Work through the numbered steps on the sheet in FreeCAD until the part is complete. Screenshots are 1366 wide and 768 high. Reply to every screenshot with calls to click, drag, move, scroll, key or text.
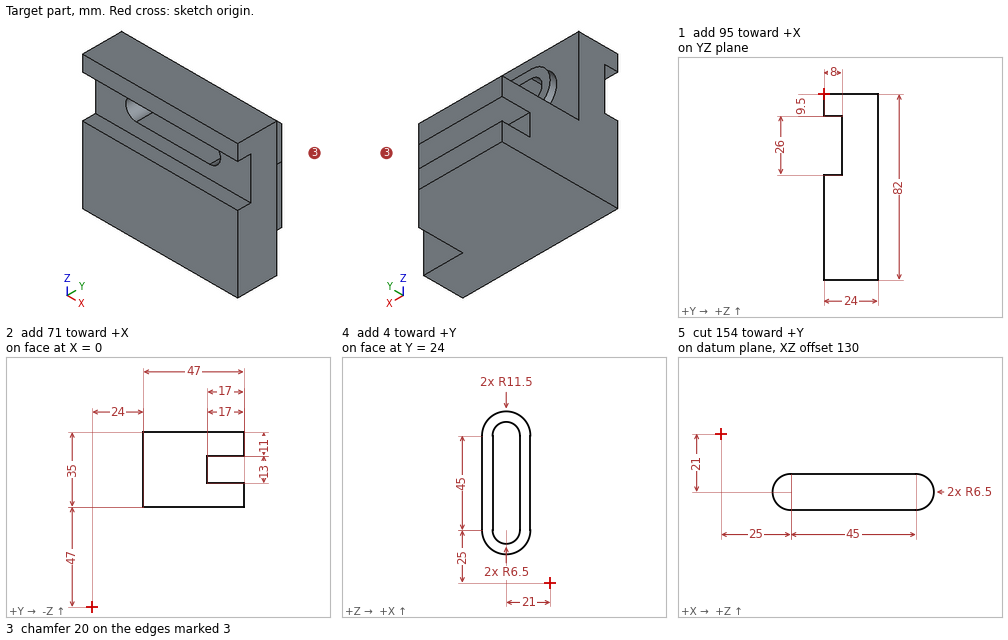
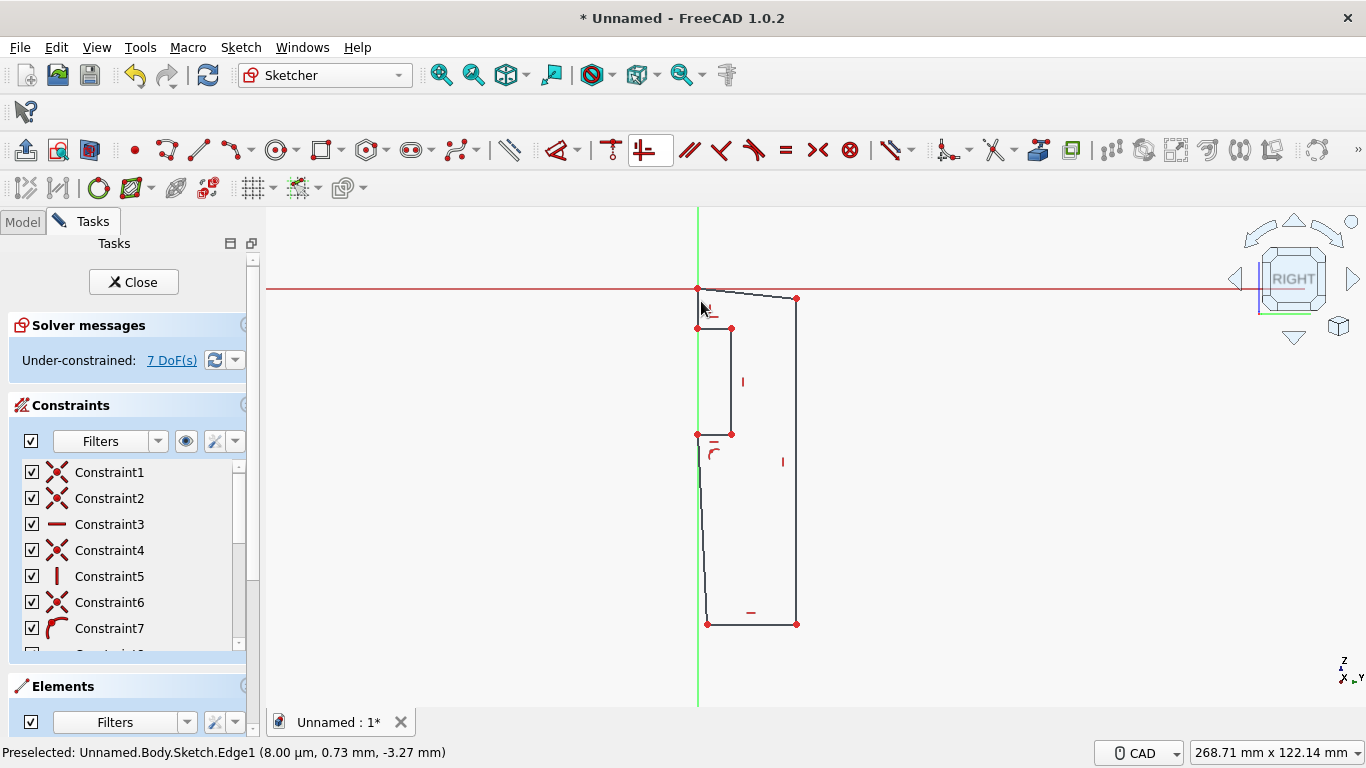
click(701, 492)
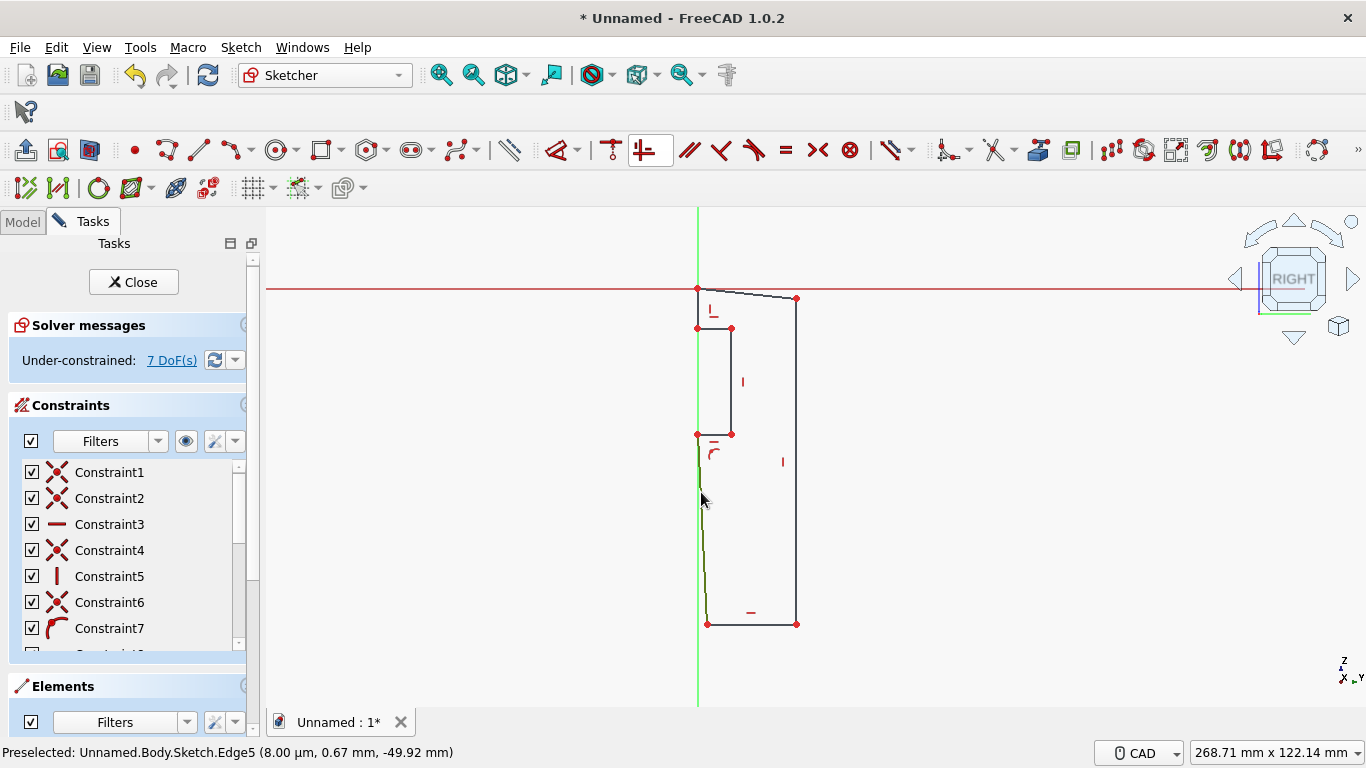
click(668, 150)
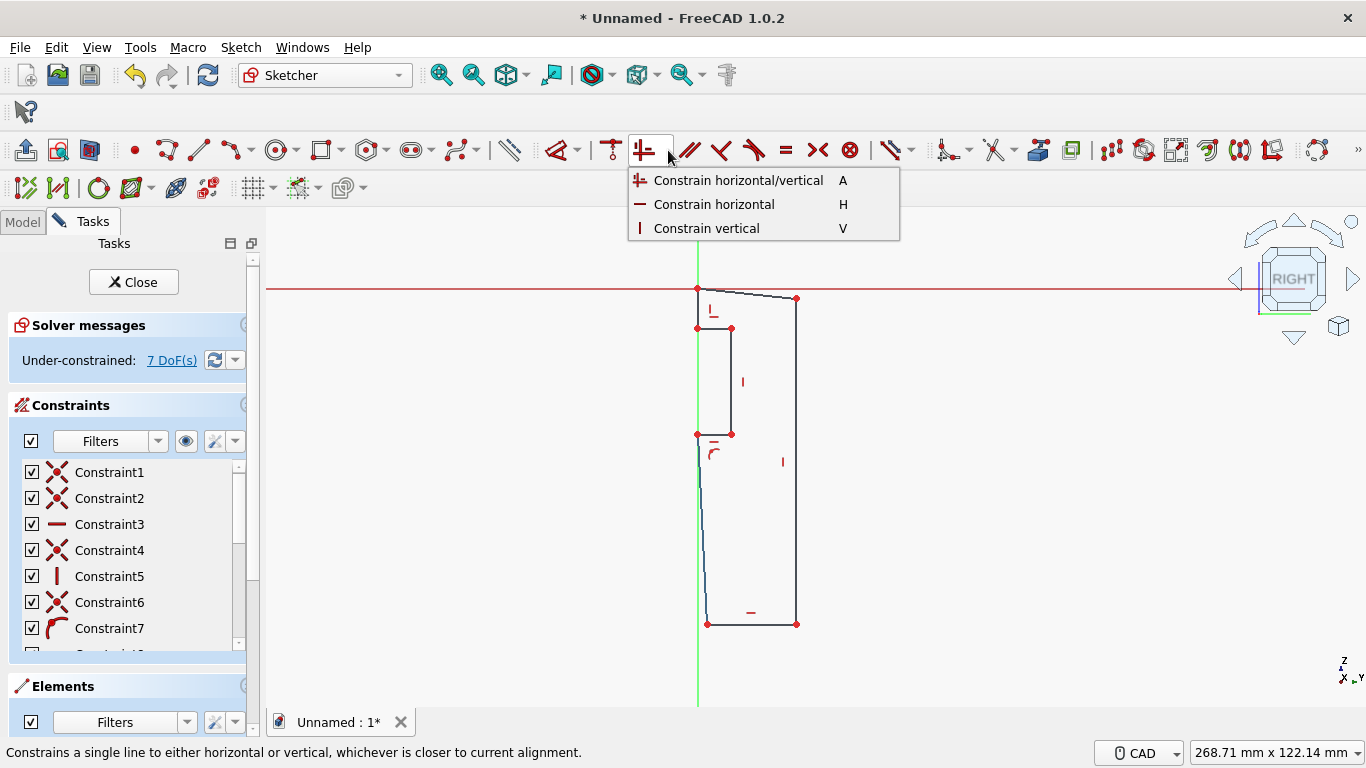
click(764, 228)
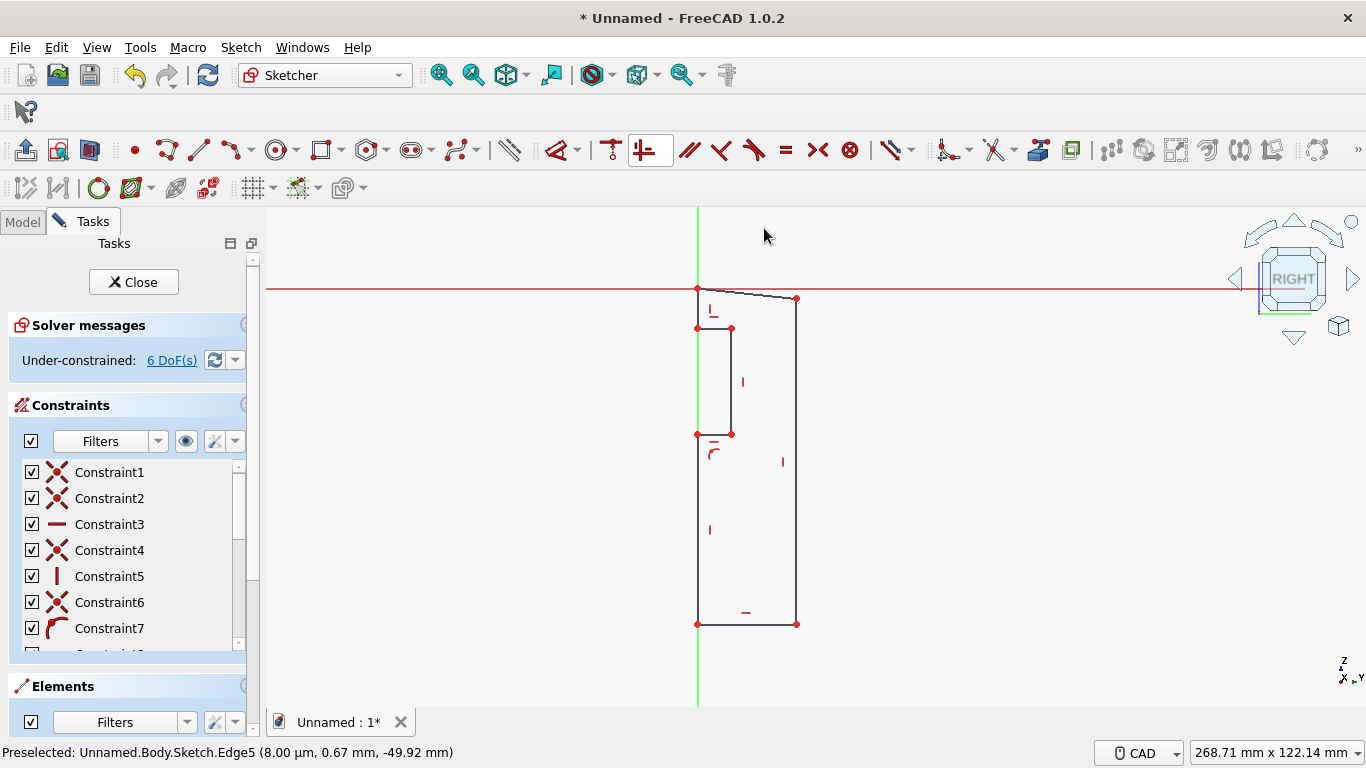
click(727, 292)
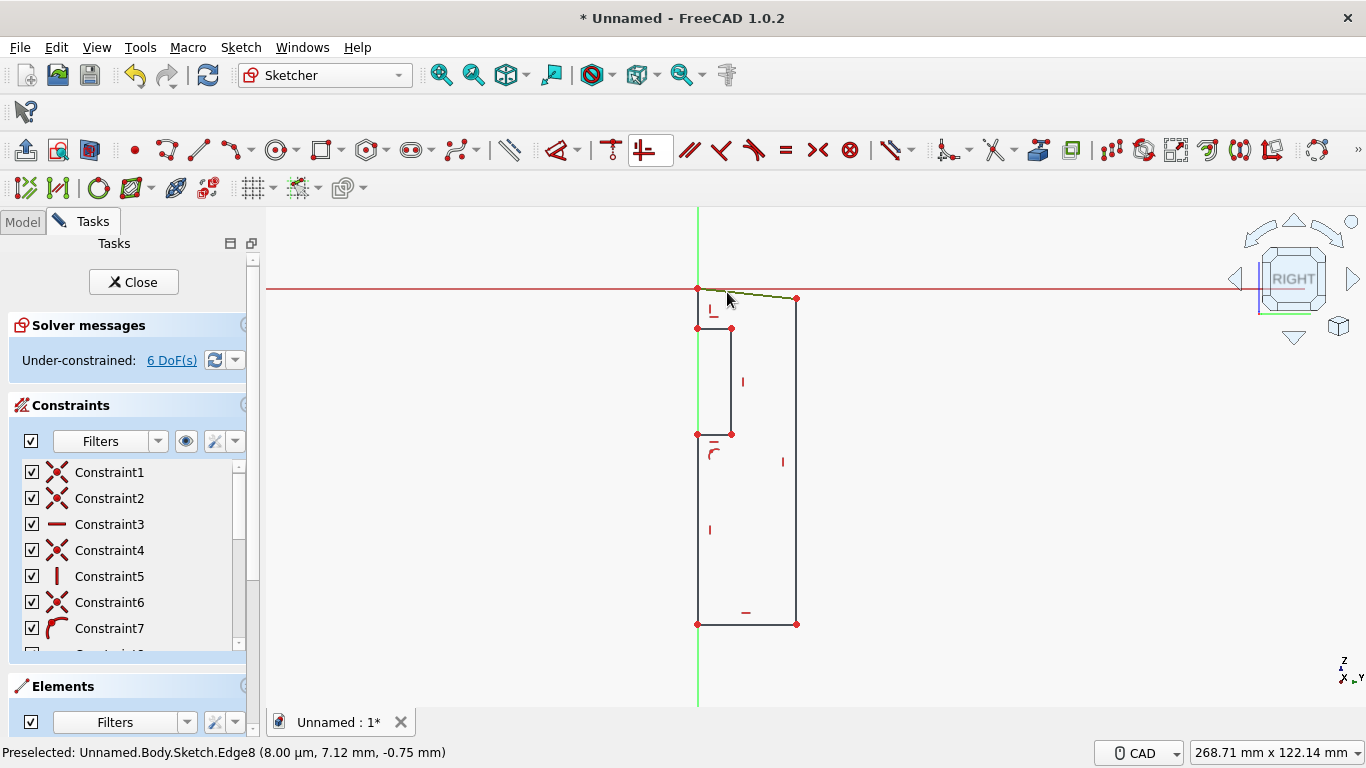
key(h)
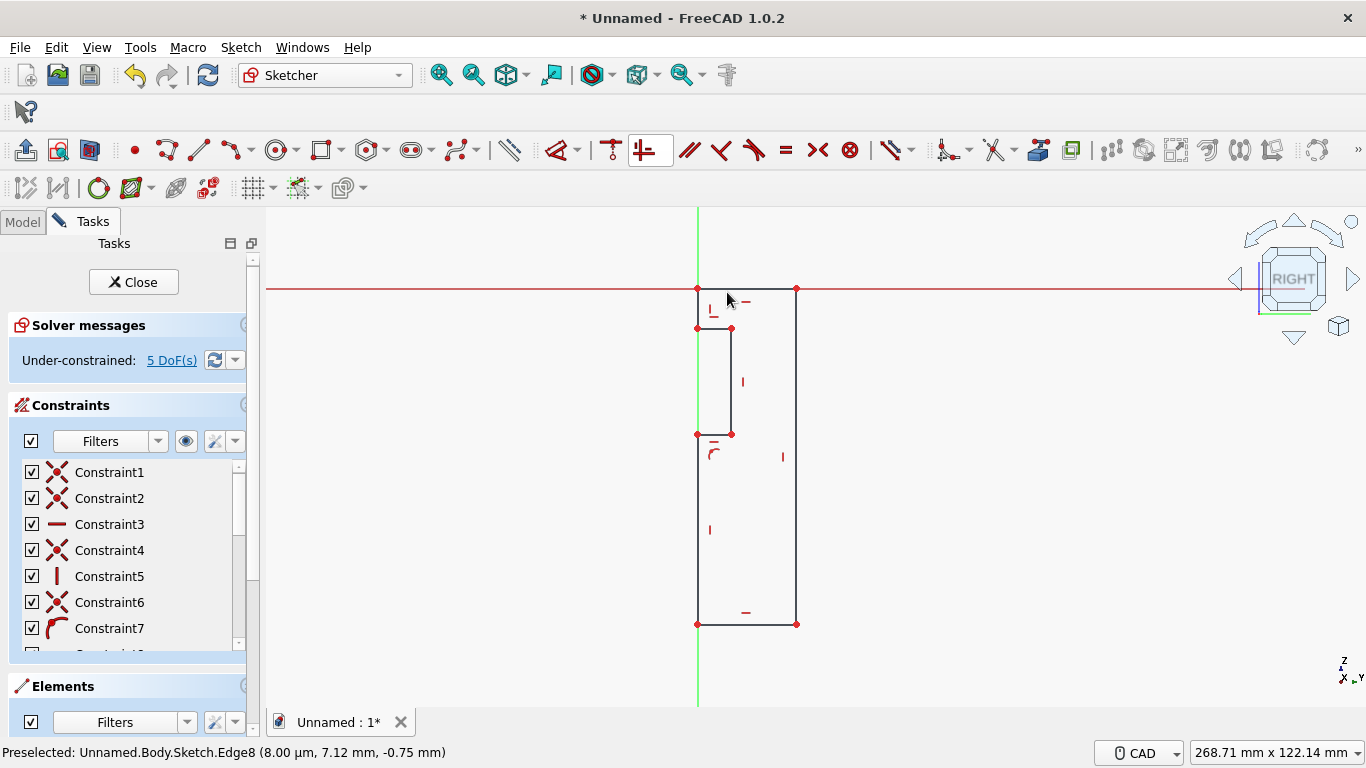
click(556, 150)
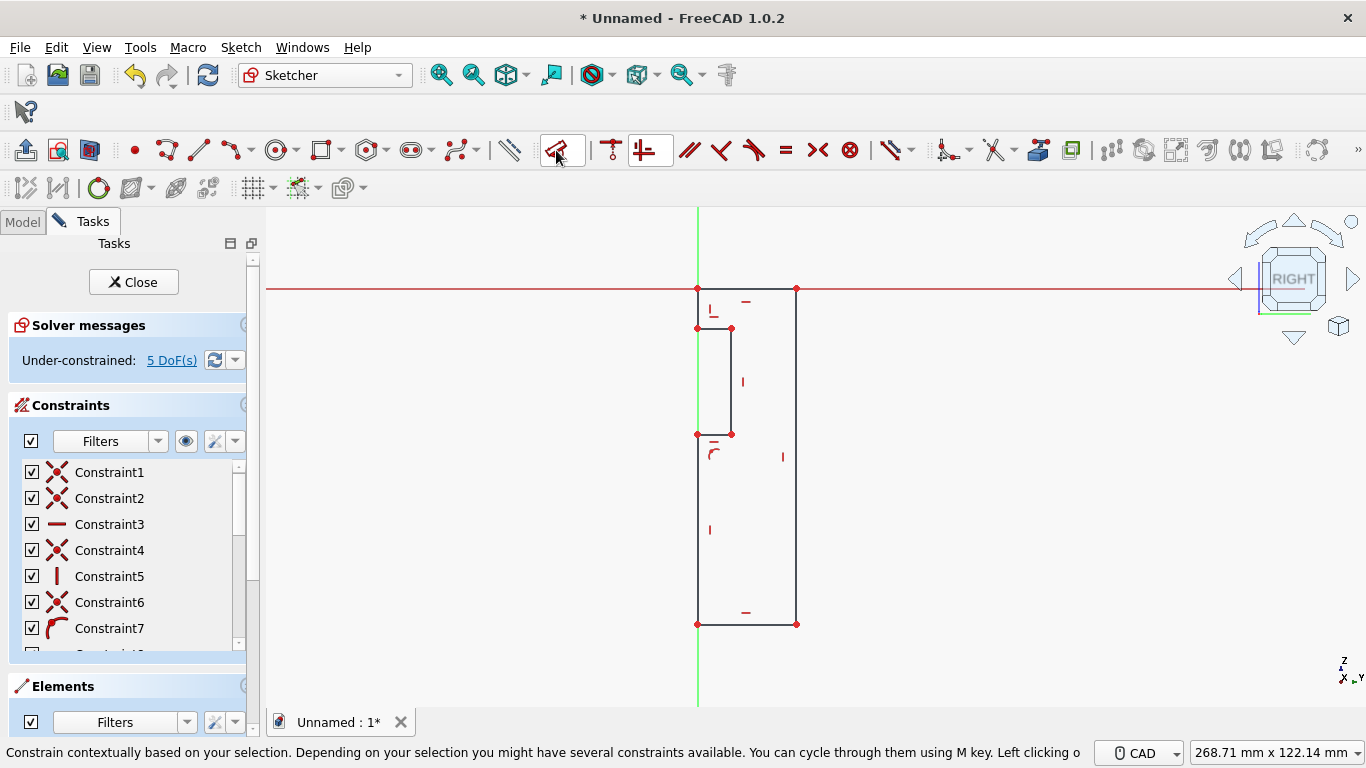
scroll(708, 329, up, 2)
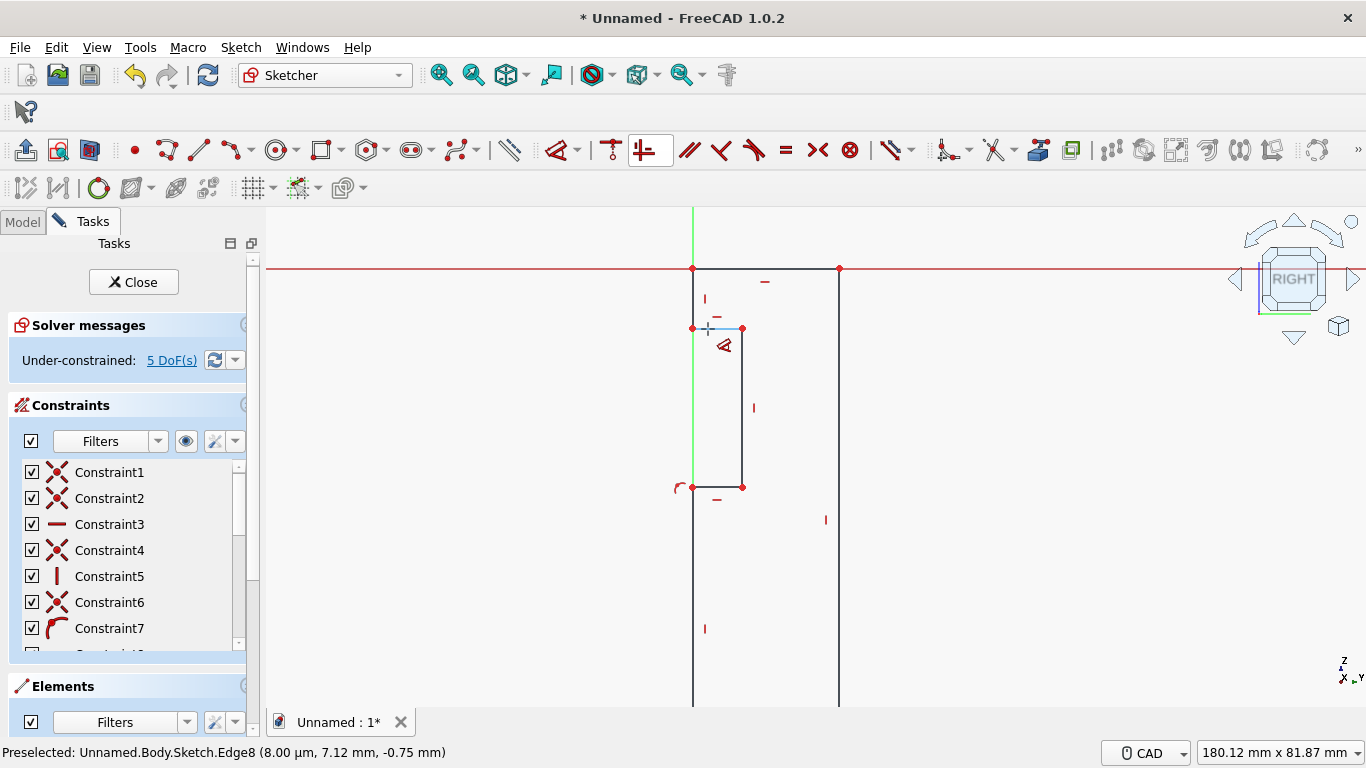
click(708, 329)
click(717, 295)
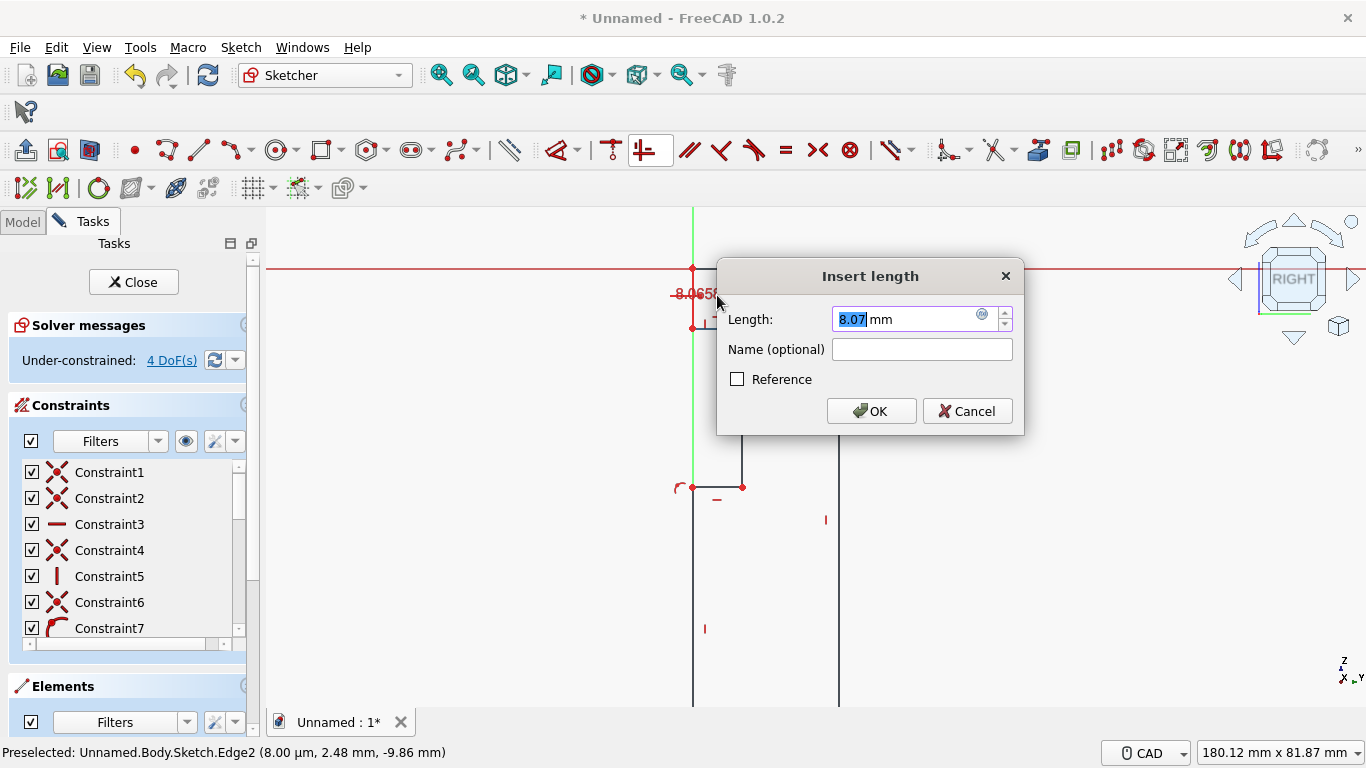
text(8)
key(Return)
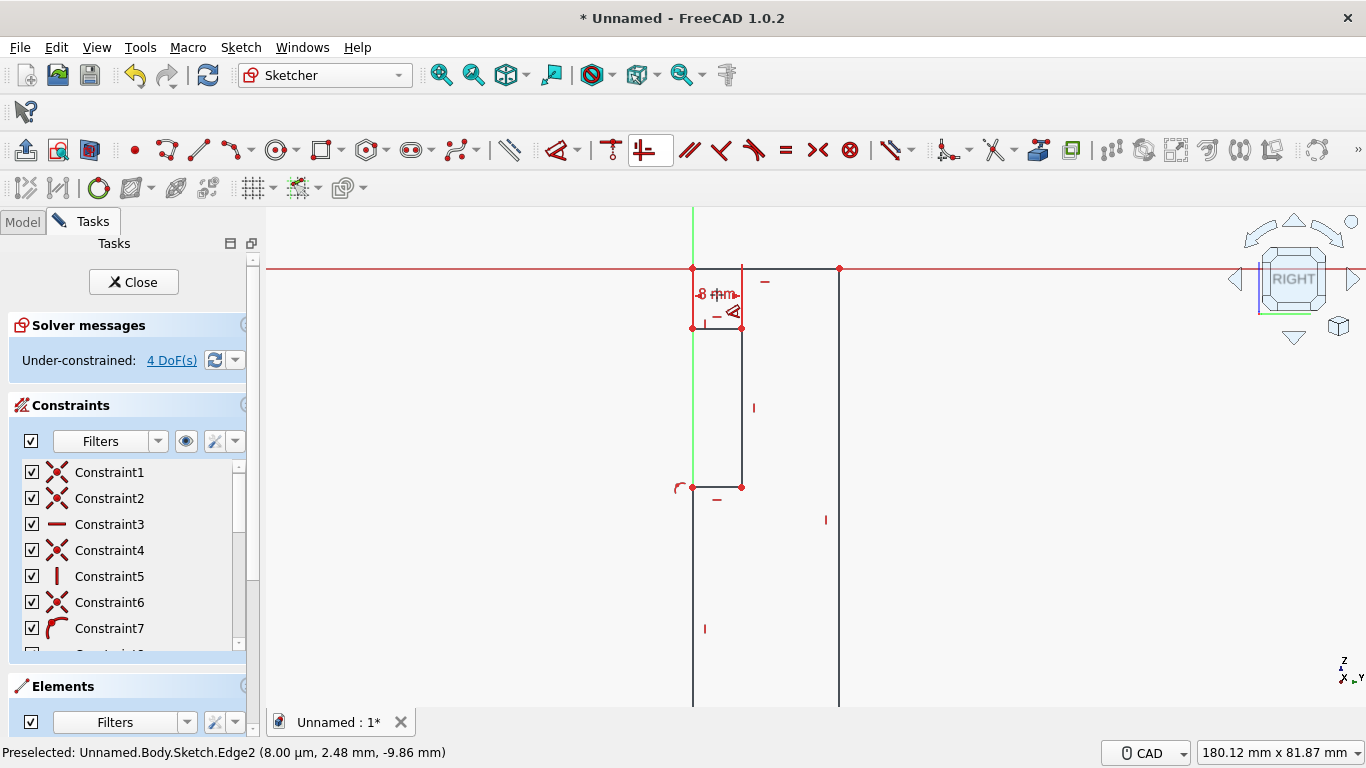
click(742, 376)
click(708, 408)